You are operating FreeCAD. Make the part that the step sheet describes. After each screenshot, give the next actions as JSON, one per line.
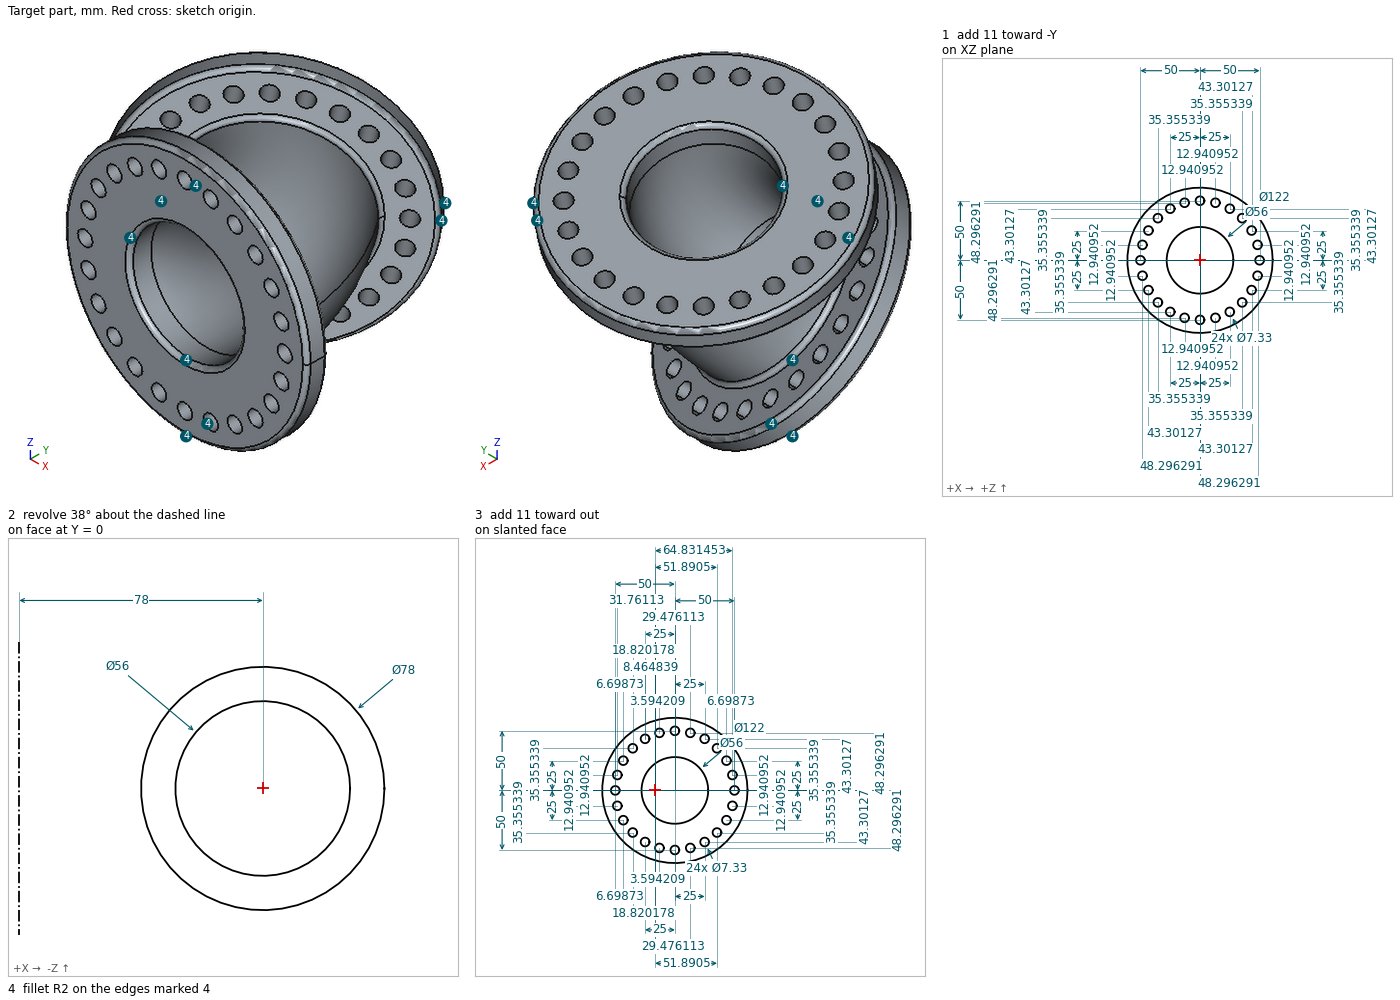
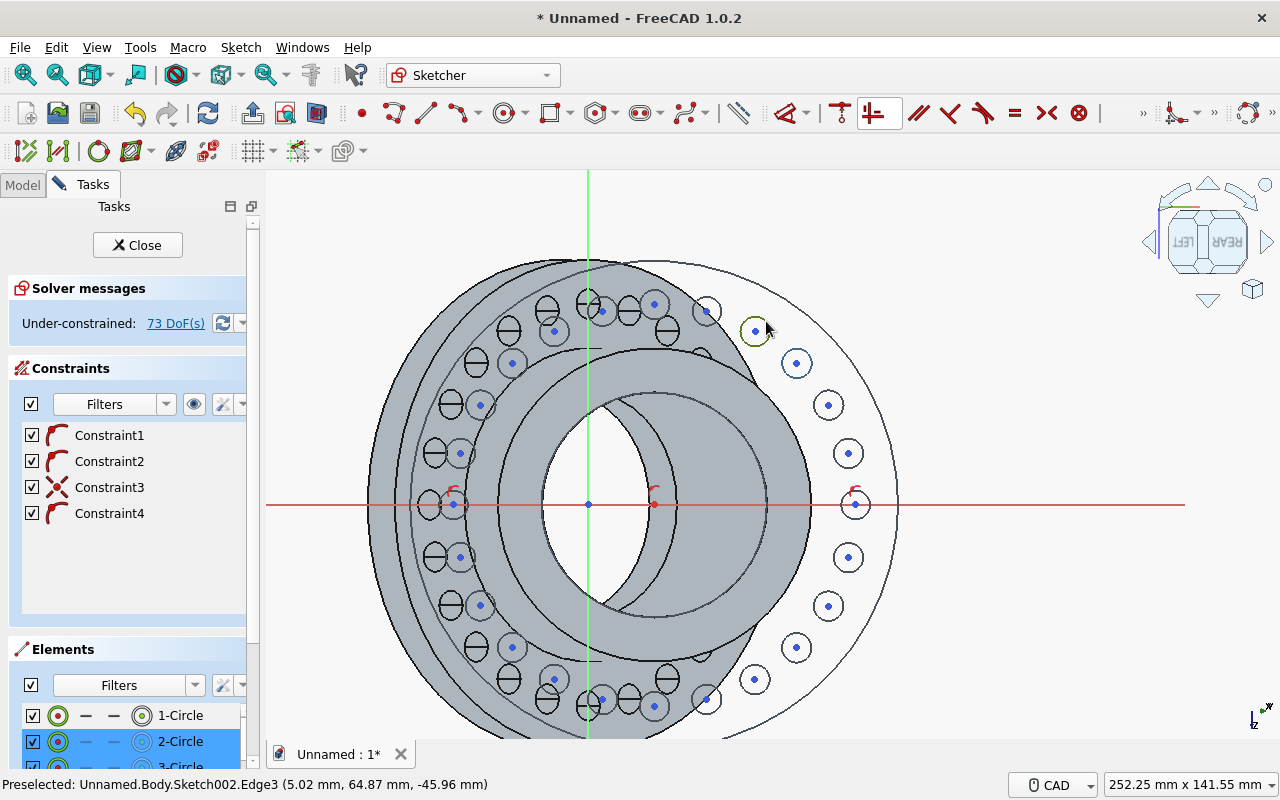
{"action": "left_click", "coordinate": [717, 301]}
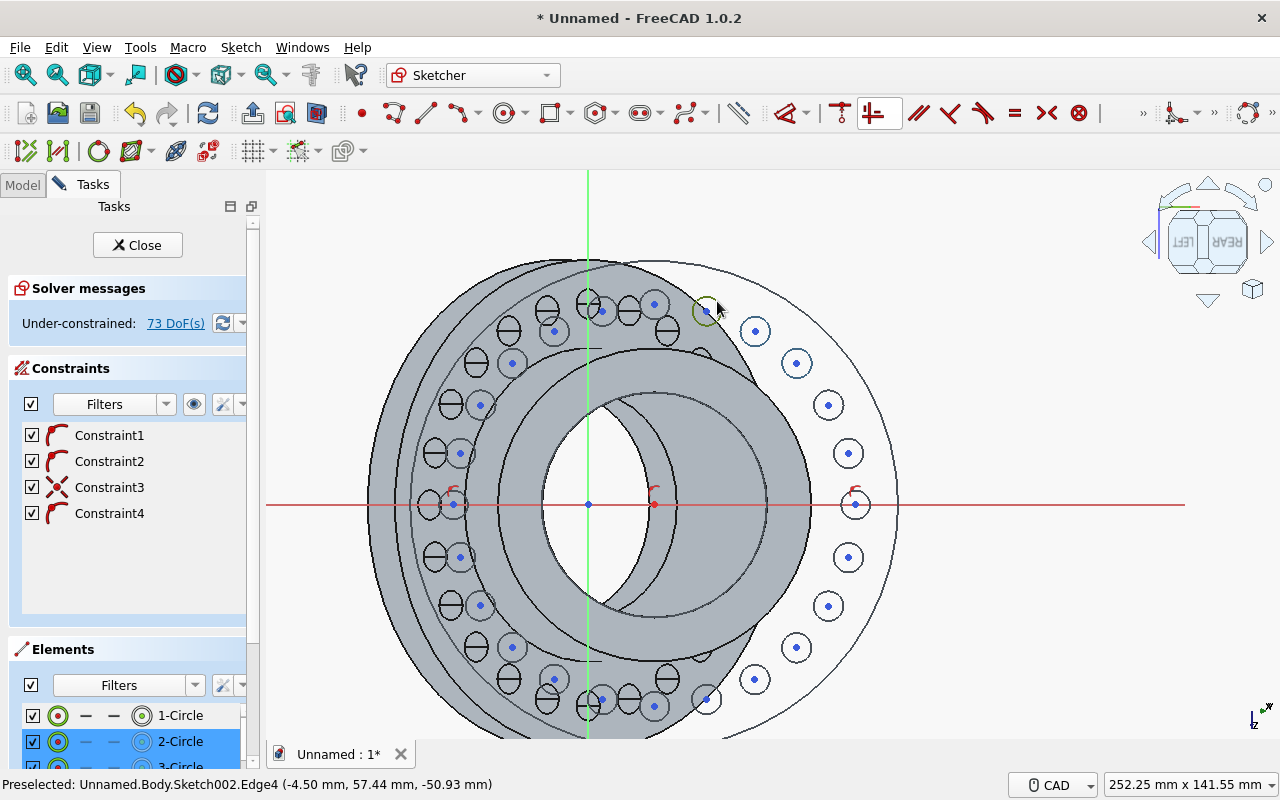
{"action": "left_click", "coordinate": [839, 395]}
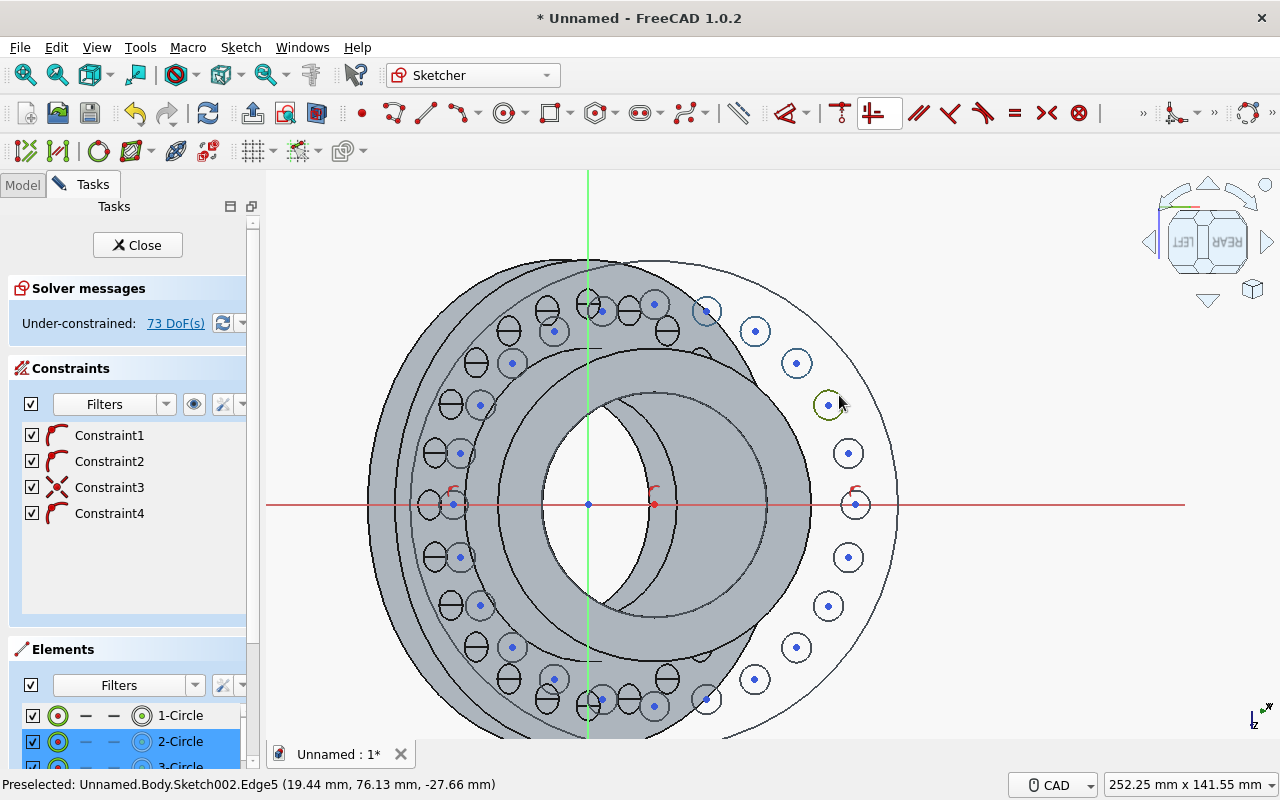
{"action": "left_click", "coordinate": [859, 443]}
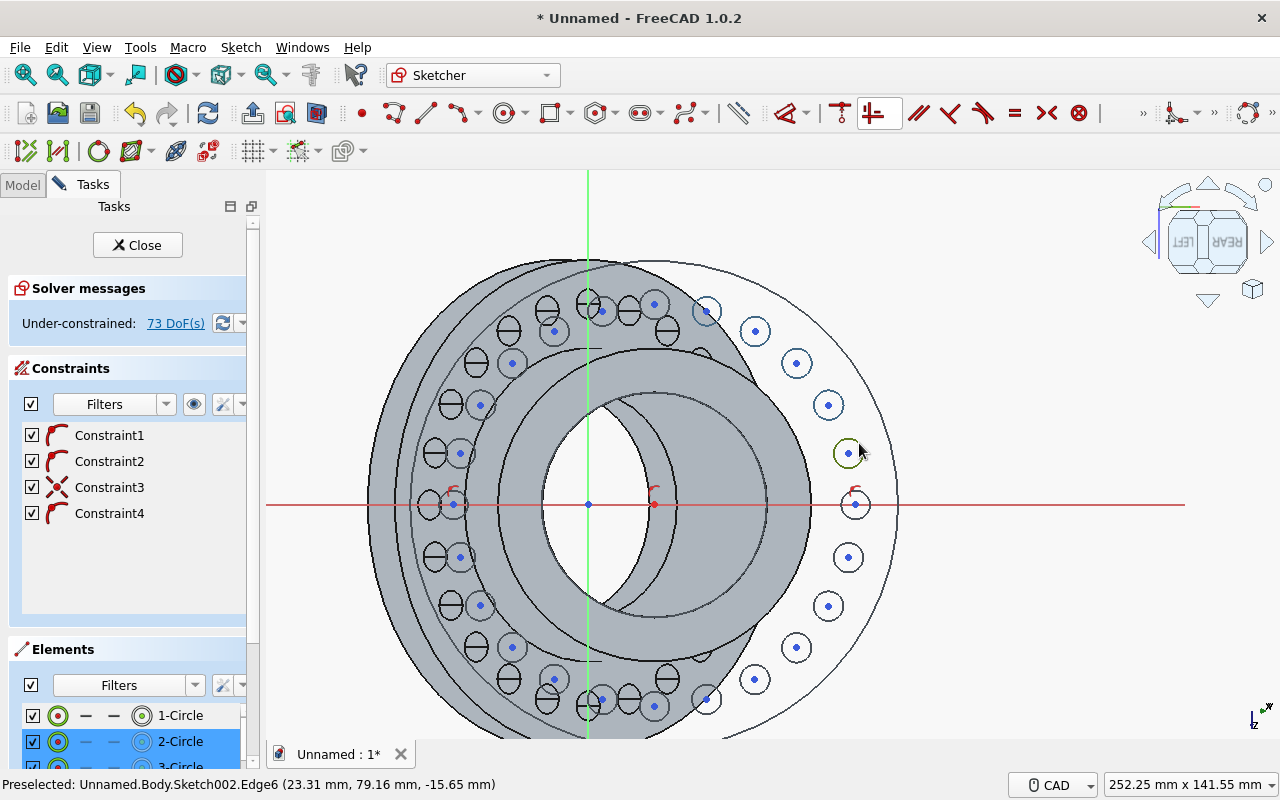
{"action": "scroll", "coordinate": [866, 495], "scroll_direction": "up", "scroll_amount": 2}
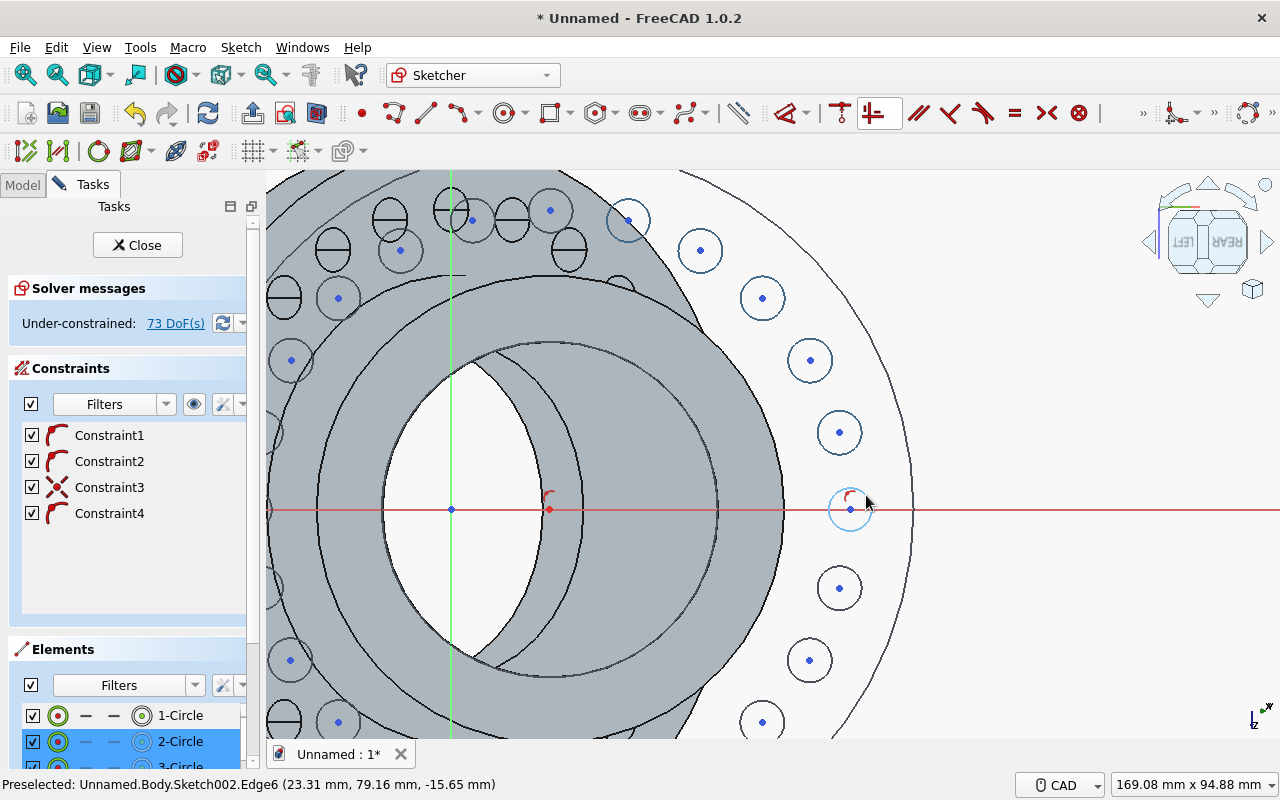
{"action": "left_click", "coordinate": [865, 494]}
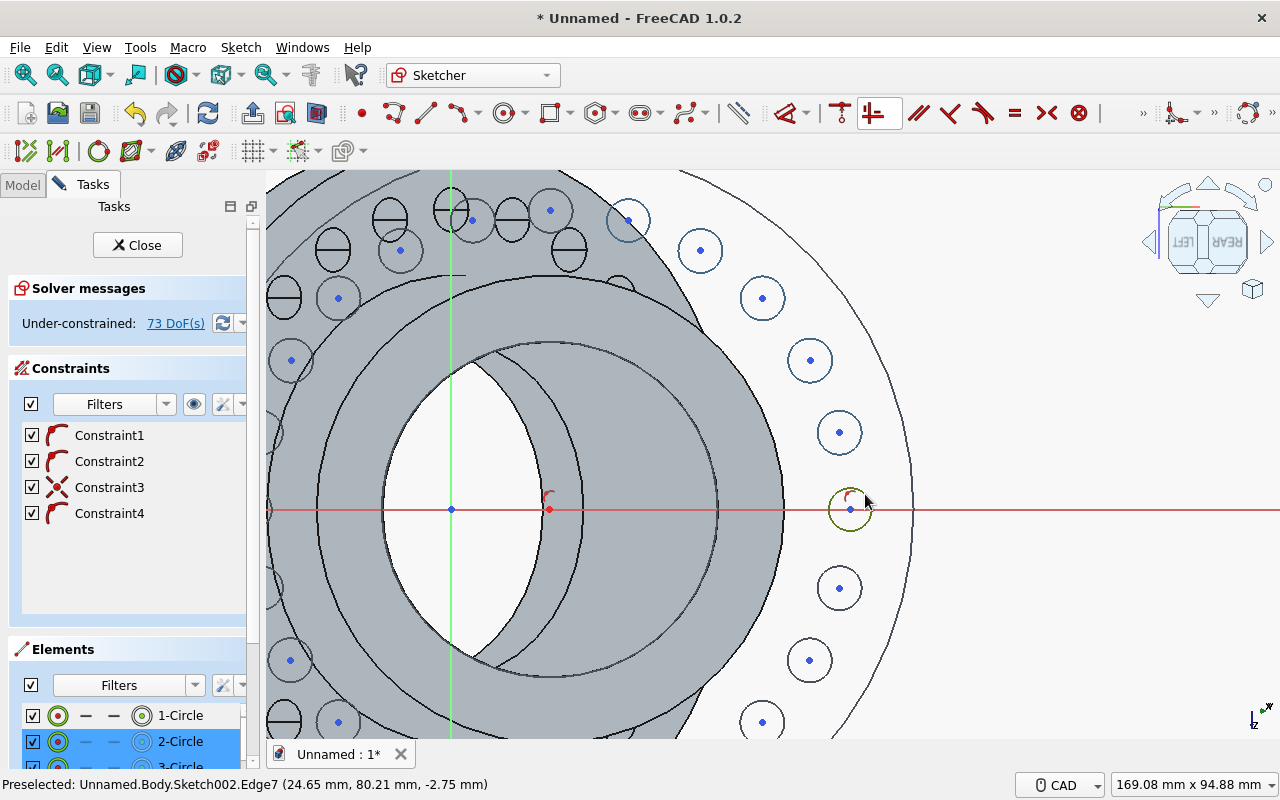
{"action": "left_click", "coordinate": [535, 226]}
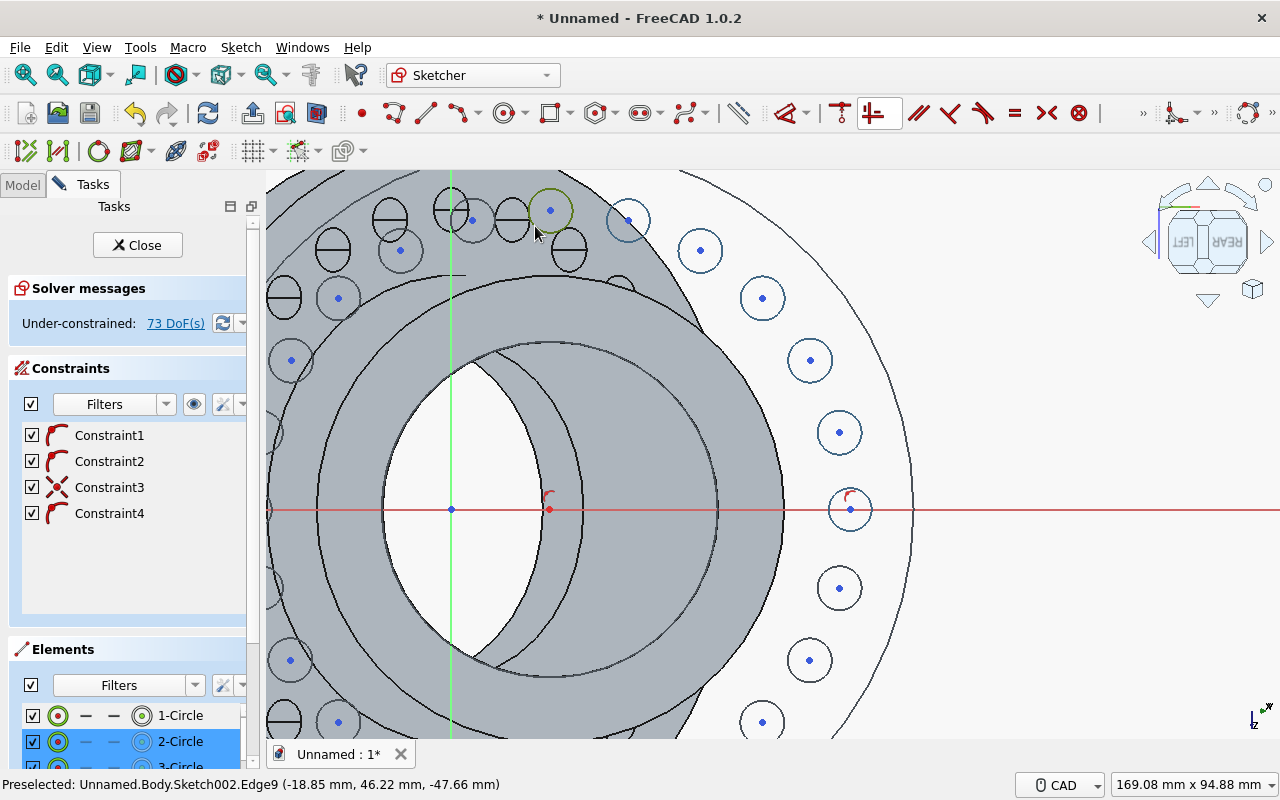
{"action": "left_click", "coordinate": [488, 205]}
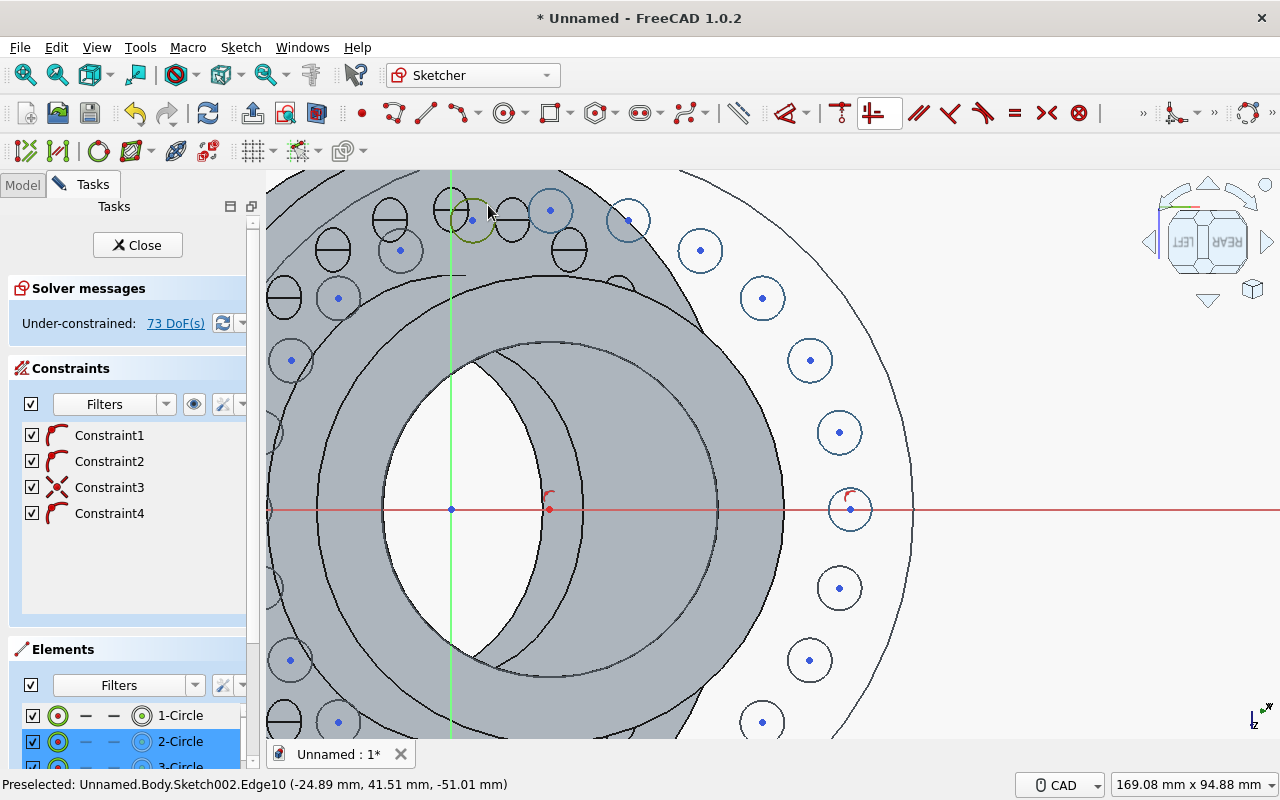
{"action": "left_click", "coordinate": [416, 235]}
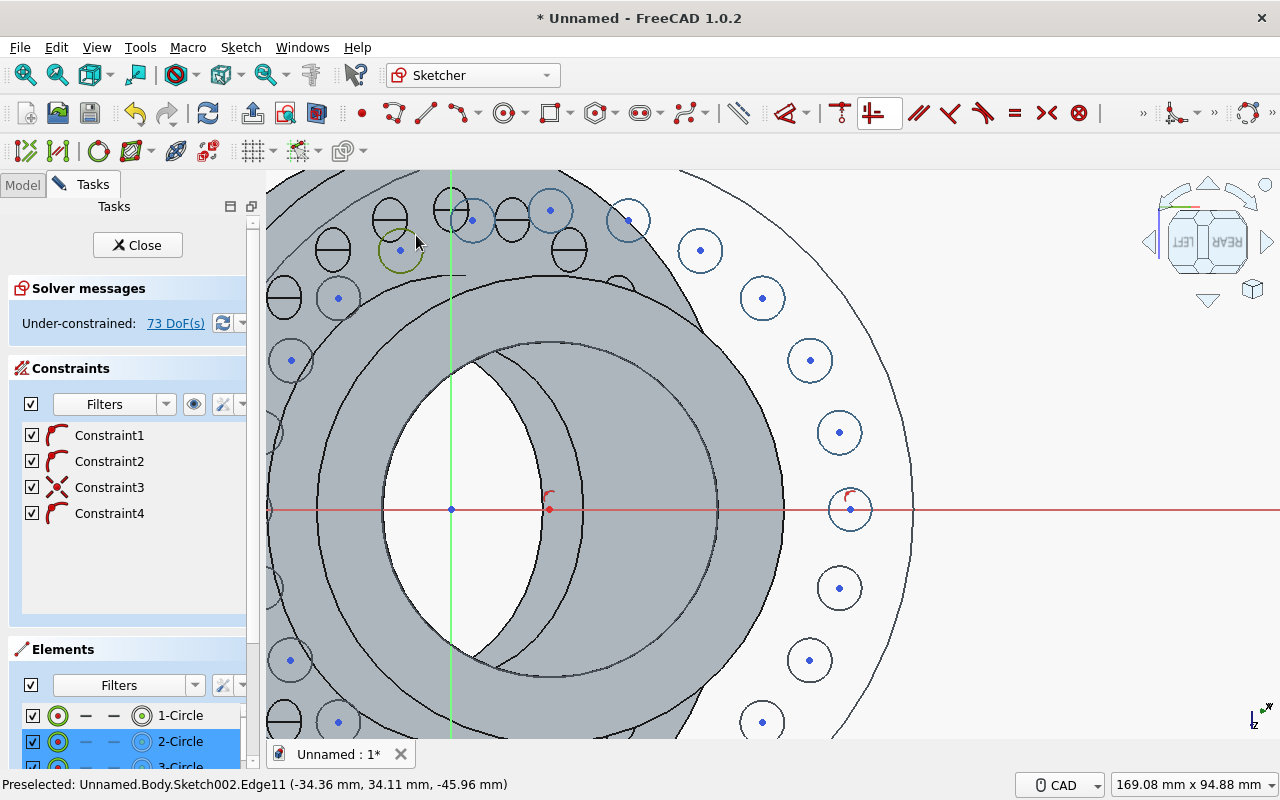
{"action": "left_click", "coordinate": [354, 283]}